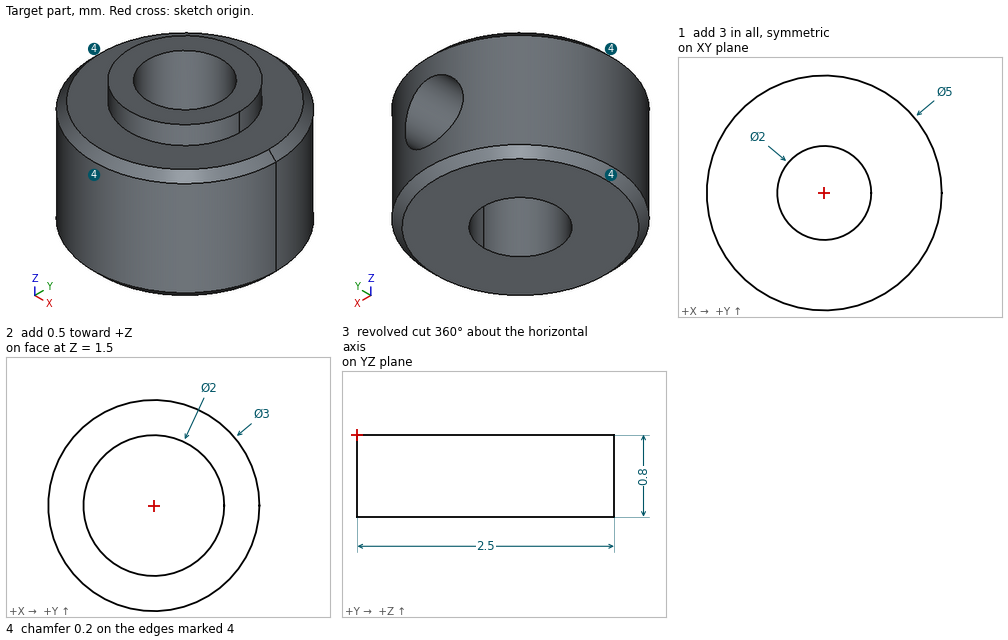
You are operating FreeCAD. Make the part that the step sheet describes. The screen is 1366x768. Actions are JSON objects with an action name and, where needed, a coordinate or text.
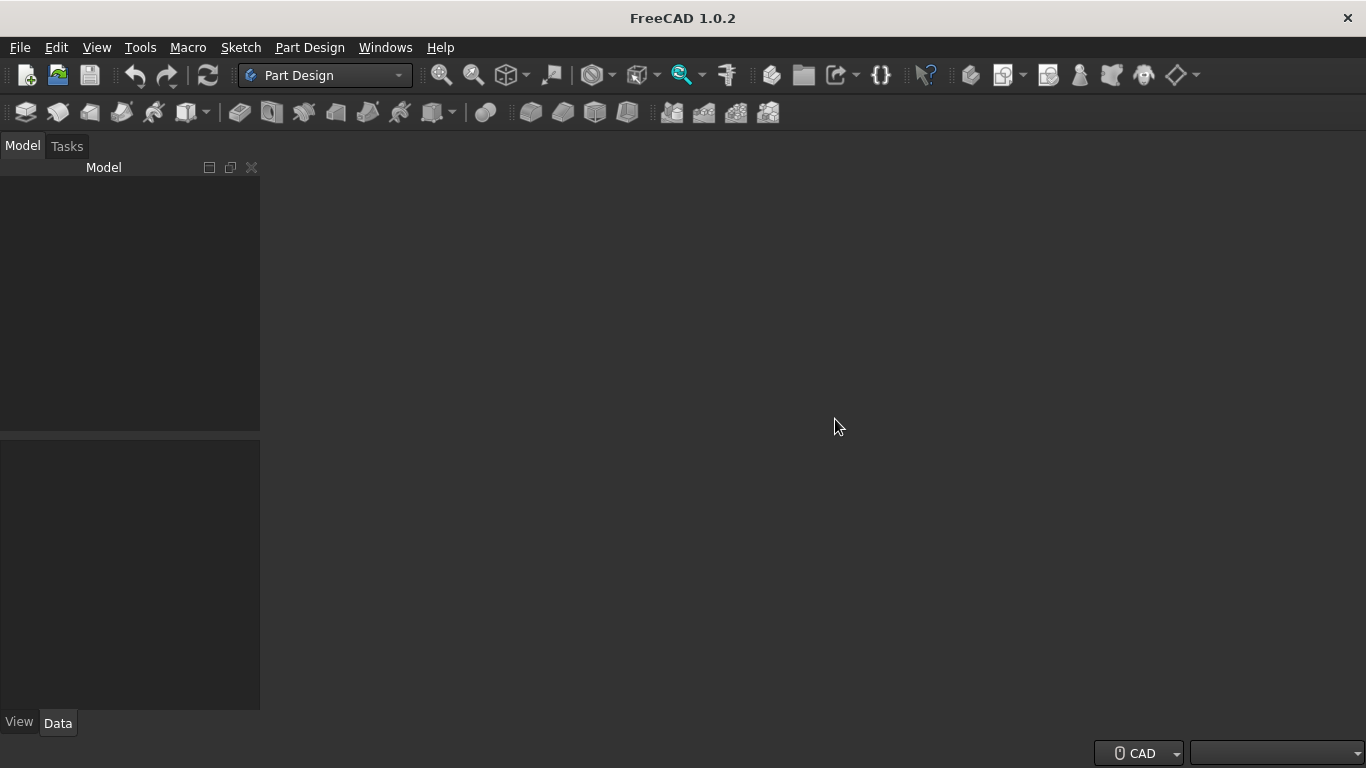
{"action": "left_click", "coordinate": [26, 76]}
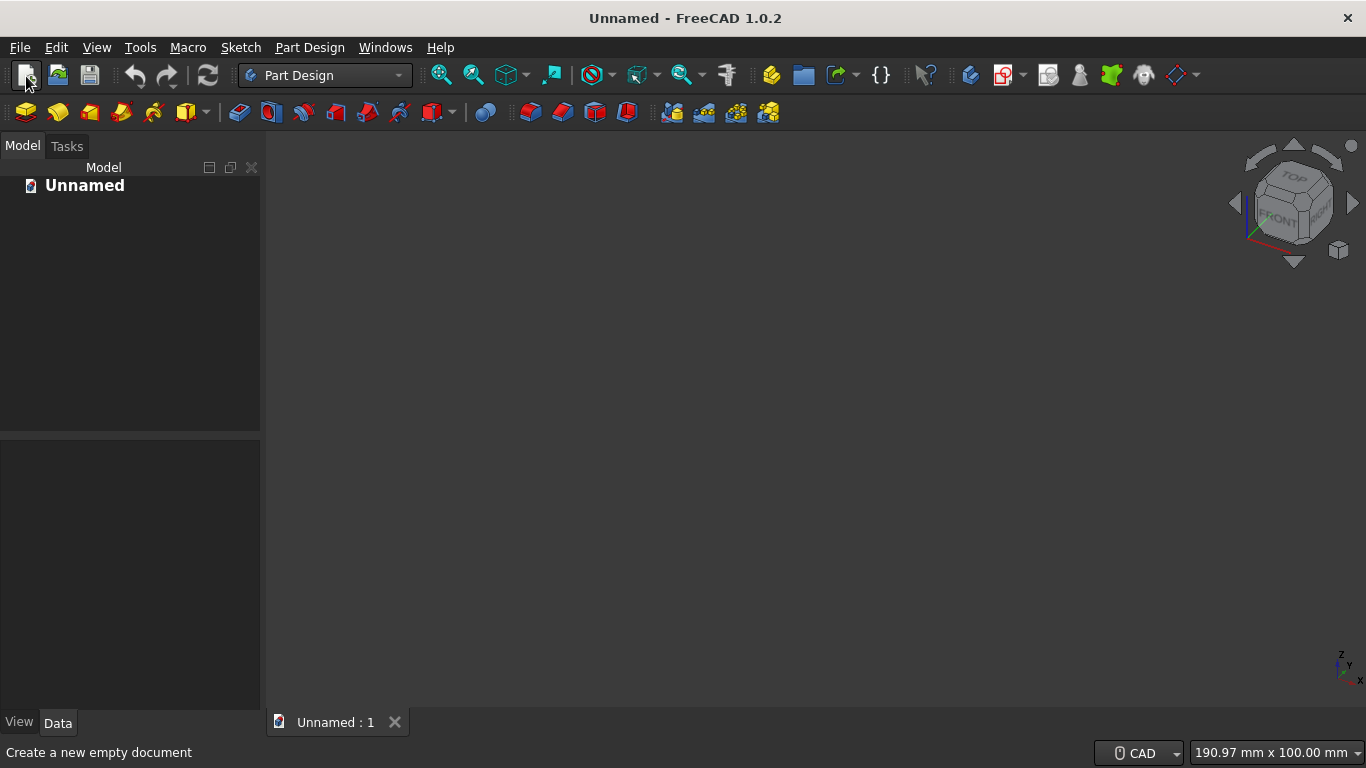
{"action": "left_click", "coordinate": [1004, 76]}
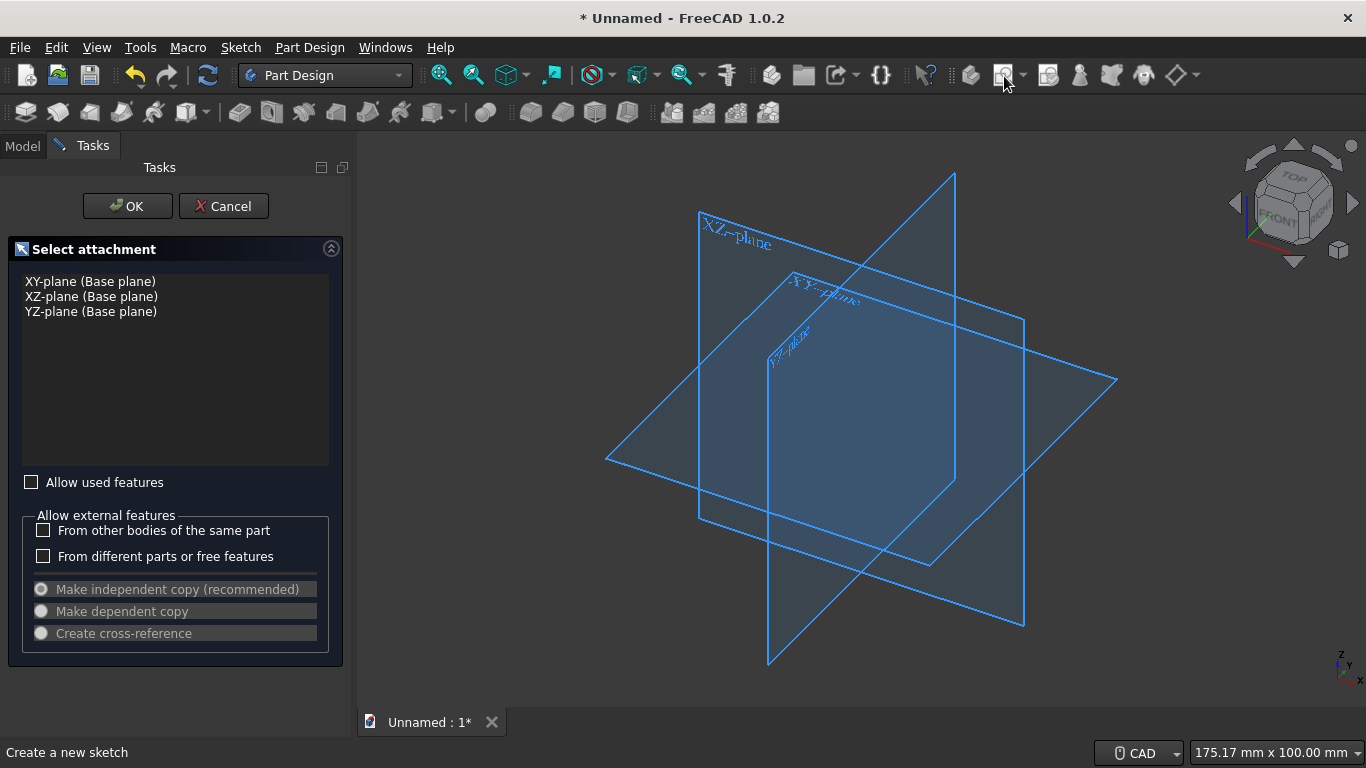
{"action": "left_click", "coordinate": [82, 282]}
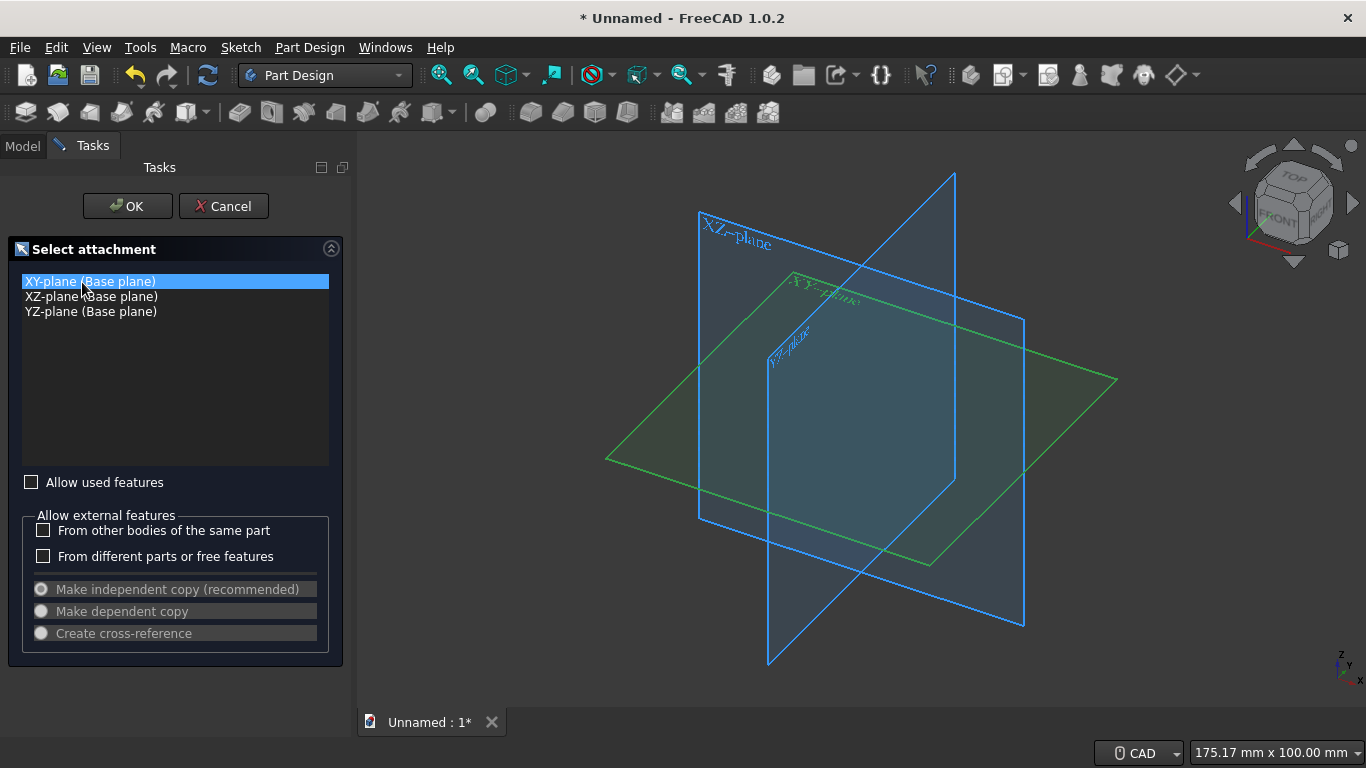
{"action": "left_click", "coordinate": [128, 206]}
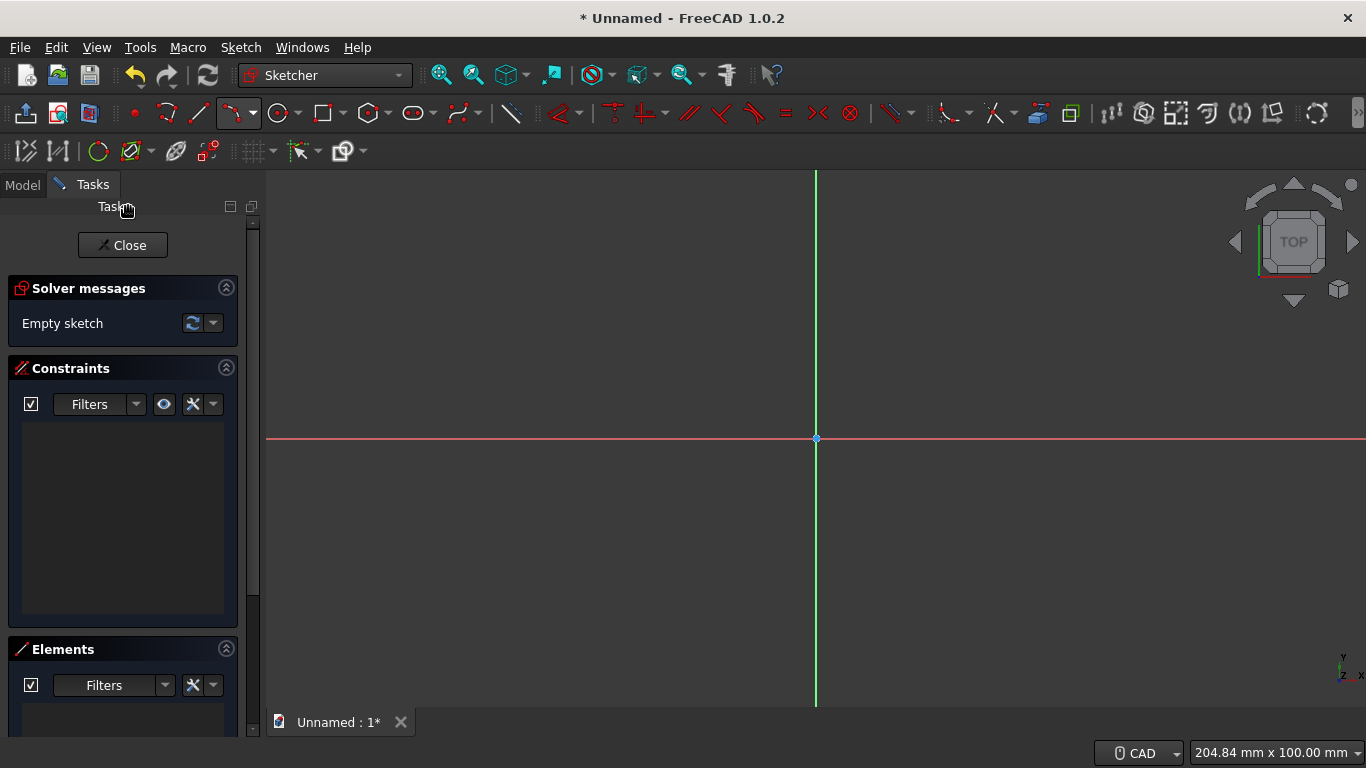
{"action": "scroll", "coordinate": [821, 438], "scroll_direction": "up", "scroll_amount": 13}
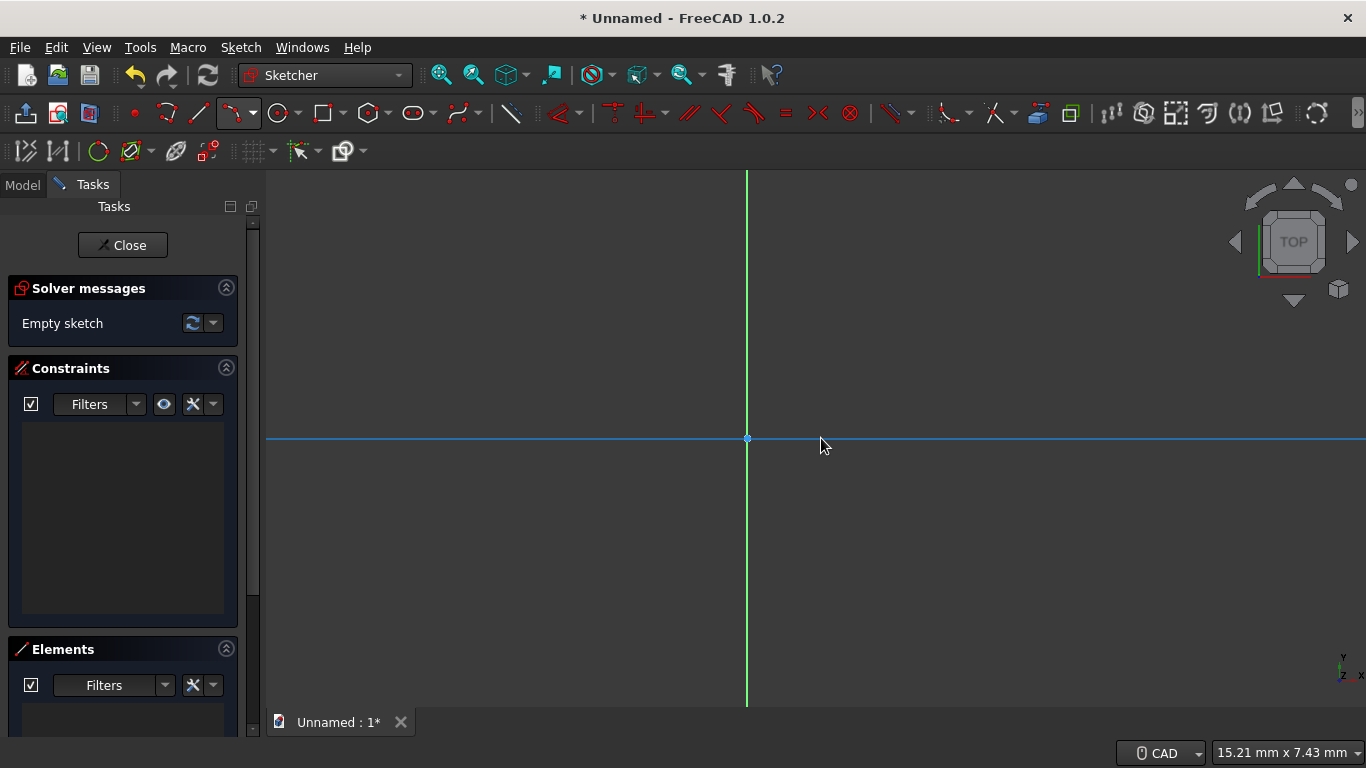
{"action": "left_click", "coordinate": [278, 114]}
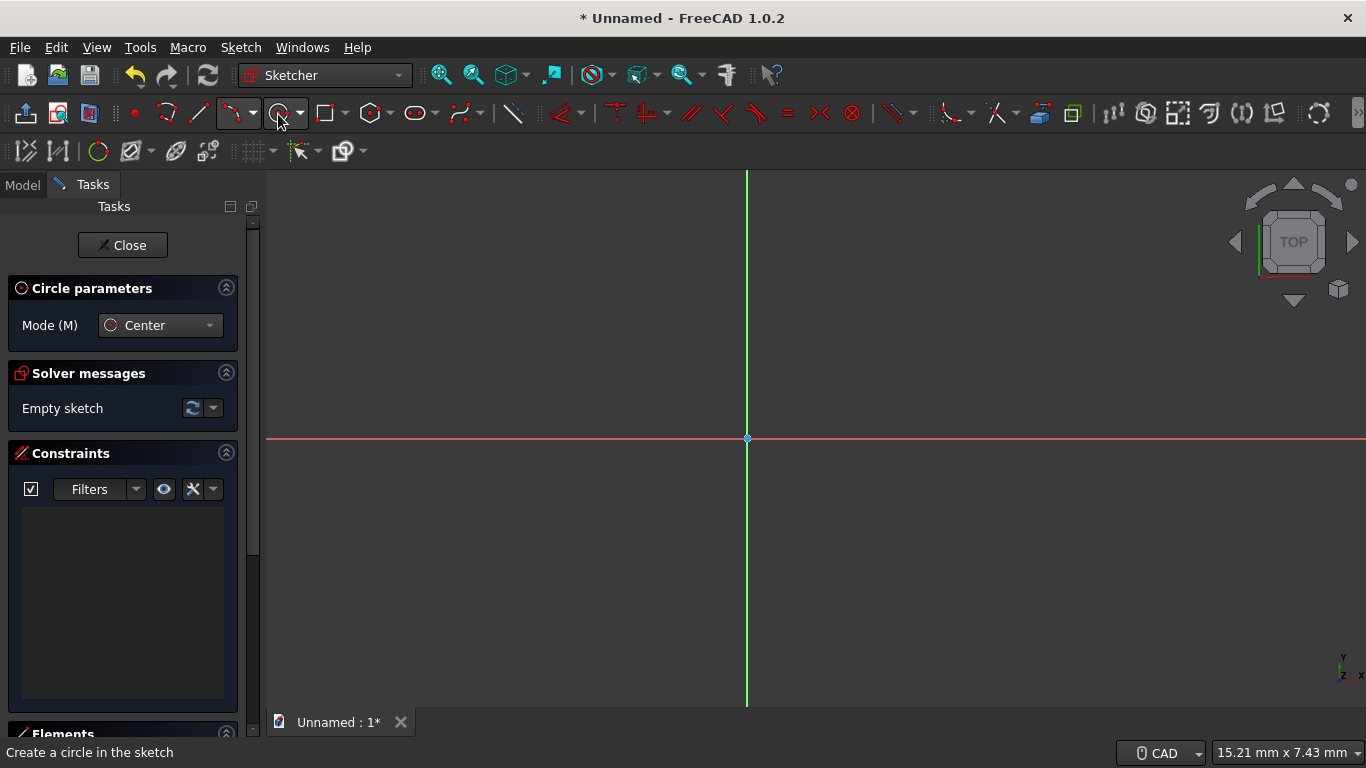
{"action": "left_click", "coordinate": [747, 438]}
{"action": "mouse_move", "coordinate": [875, 311]}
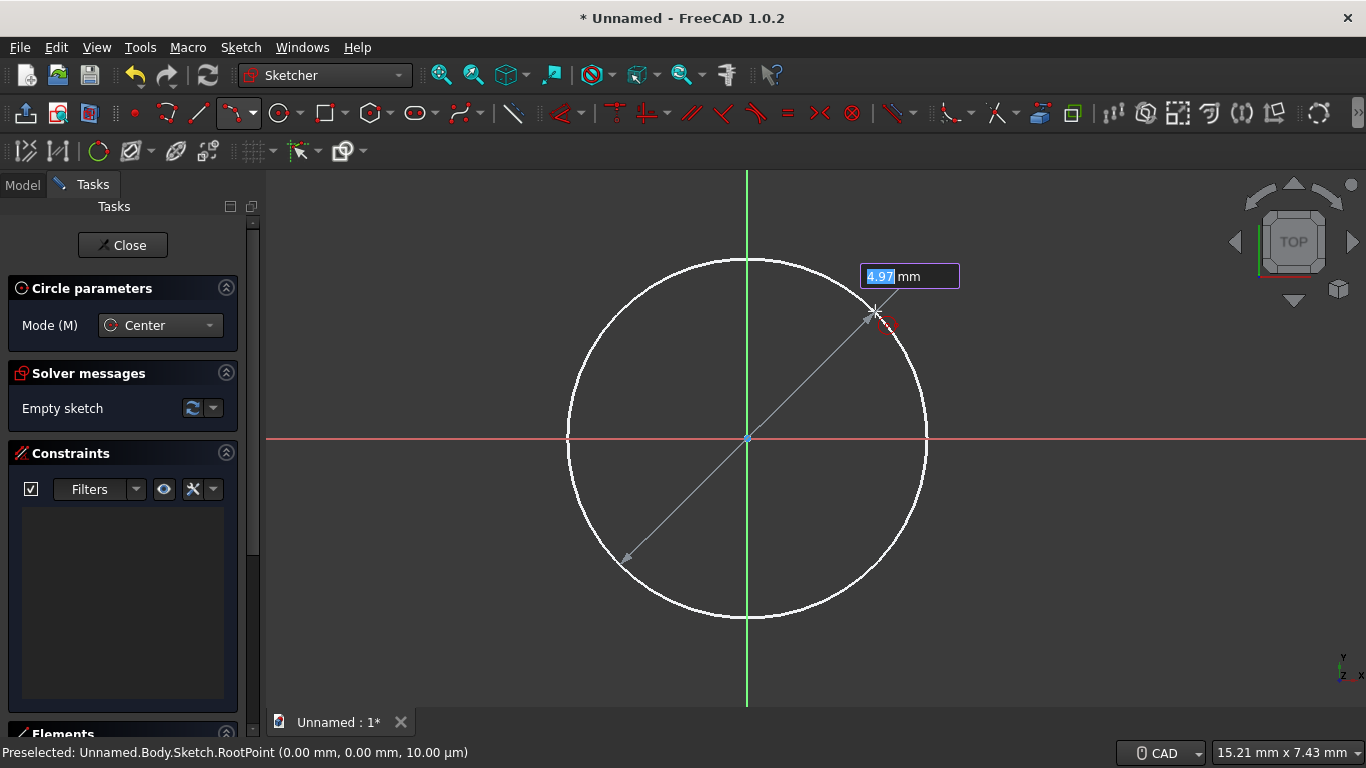
{"action": "type", "text": "5"}
{"action": "key", "text": "Return"}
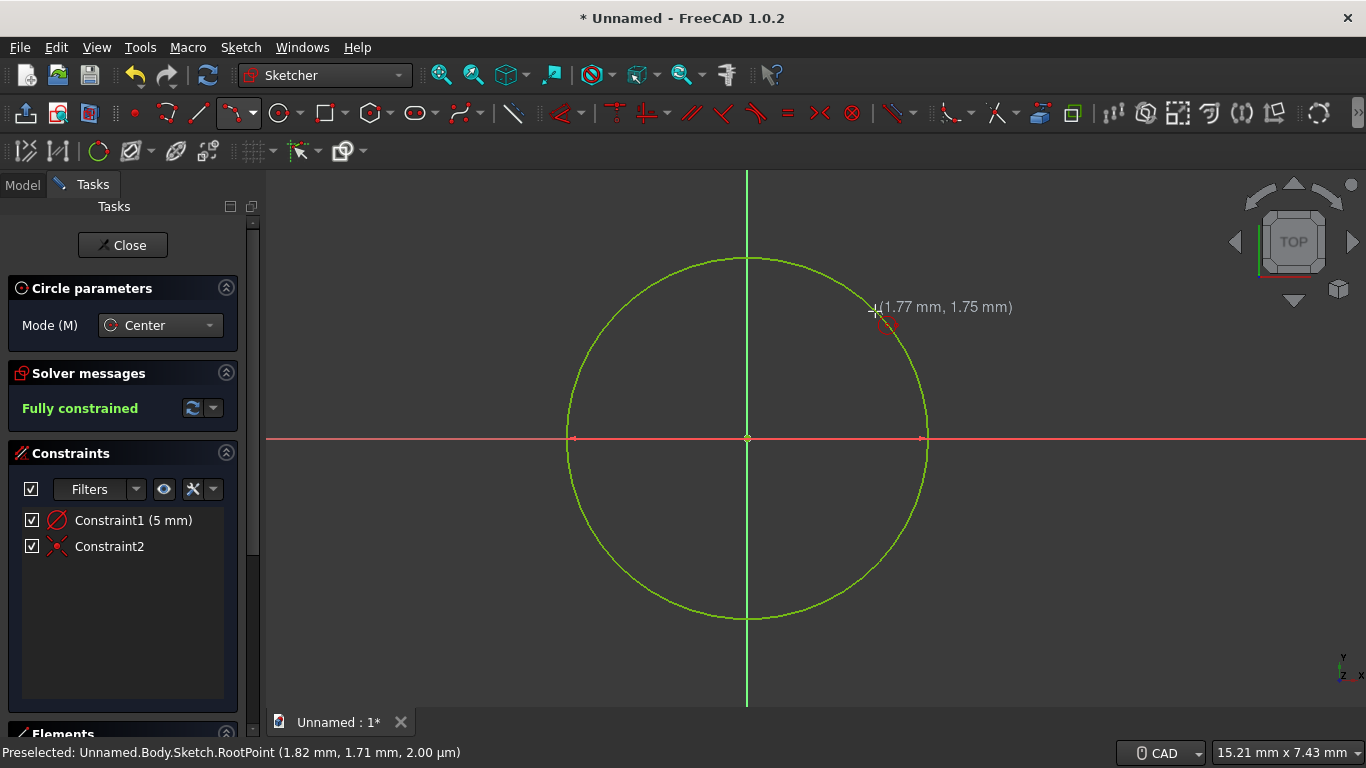
{"action": "left_click", "coordinate": [747, 438]}
{"action": "mouse_move", "coordinate": [799, 387]}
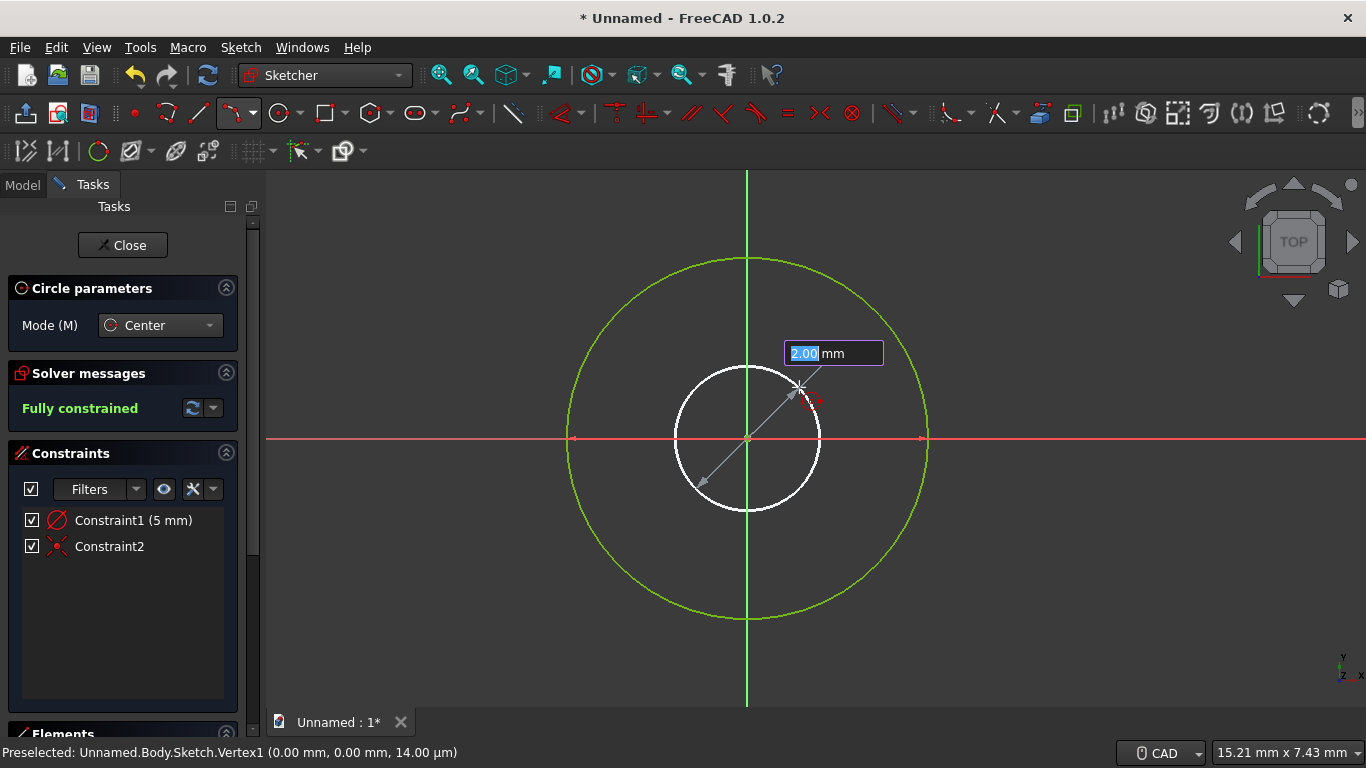
{"action": "type", "text": "2"}
{"action": "key", "text": "Return"}
{"action": "key", "text": "Escape"}